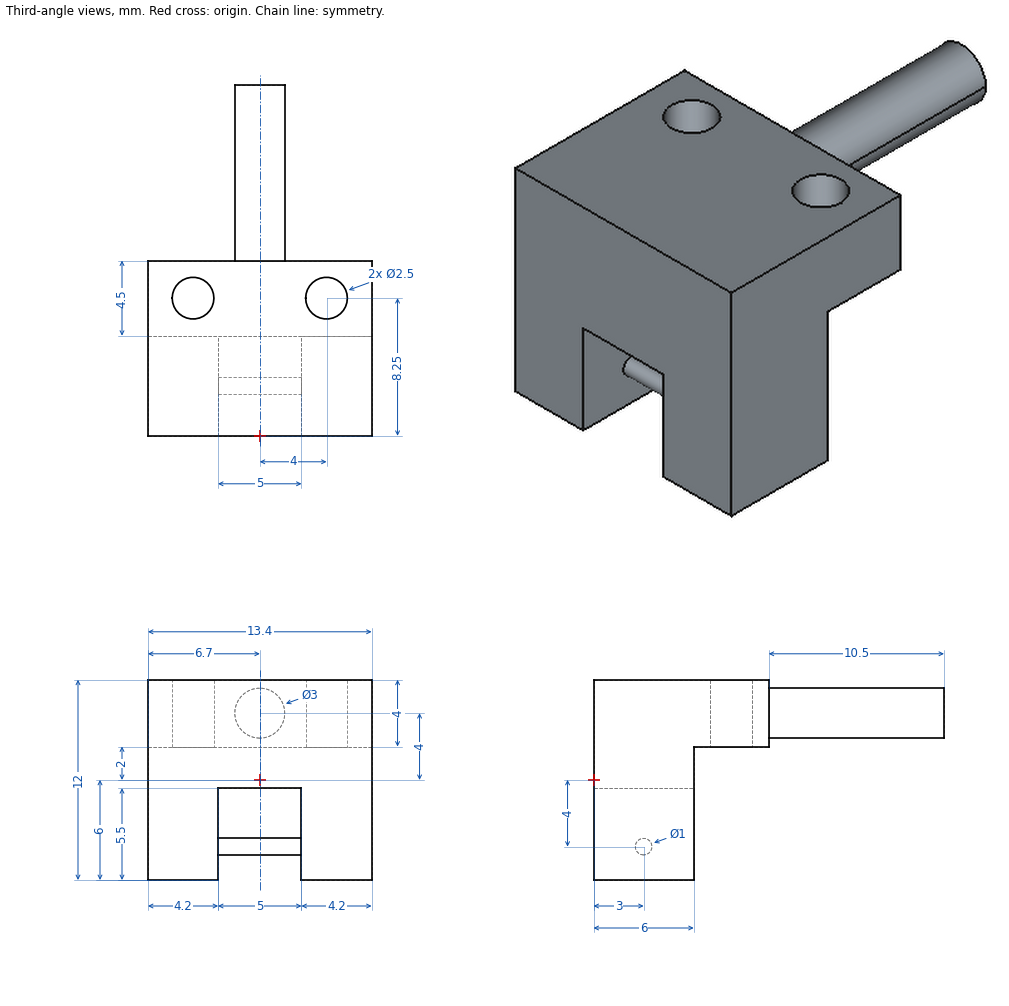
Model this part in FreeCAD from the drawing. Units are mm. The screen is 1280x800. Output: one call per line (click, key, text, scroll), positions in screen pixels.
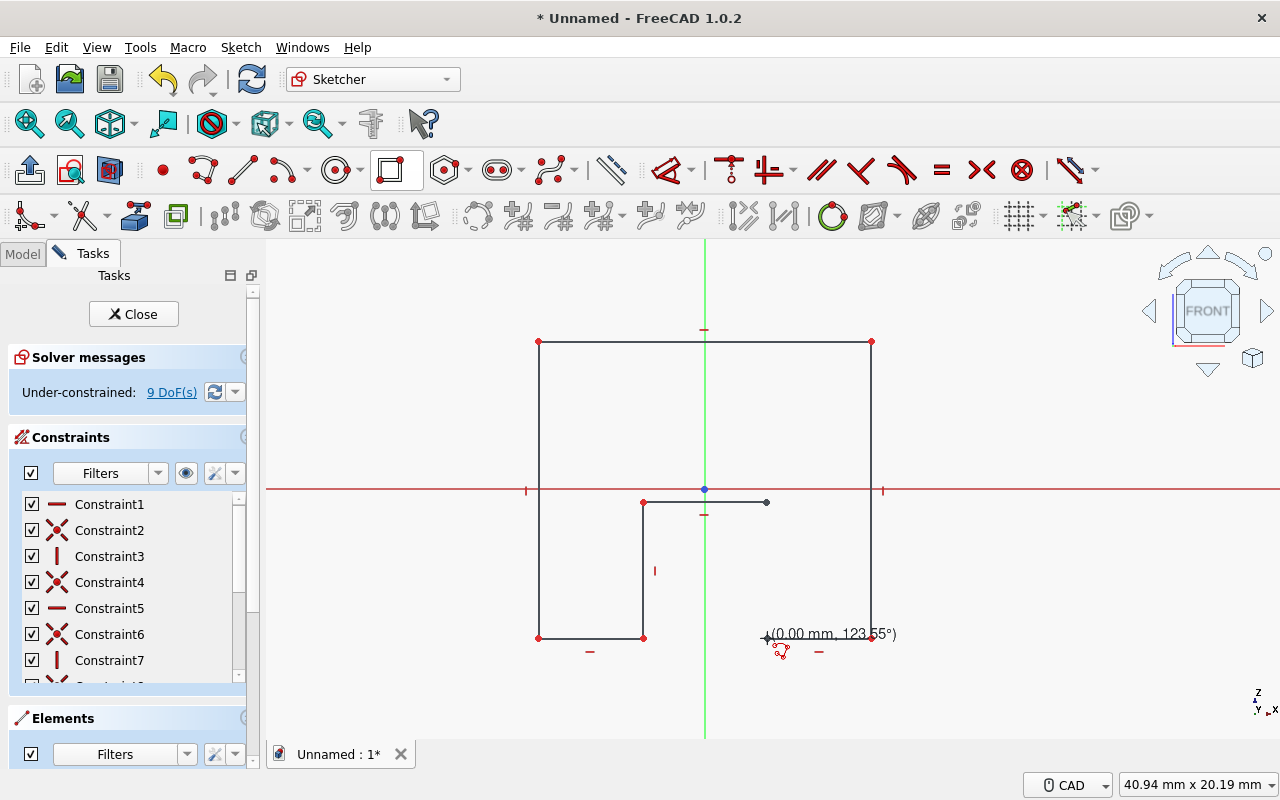
scroll(767, 502, up, 2)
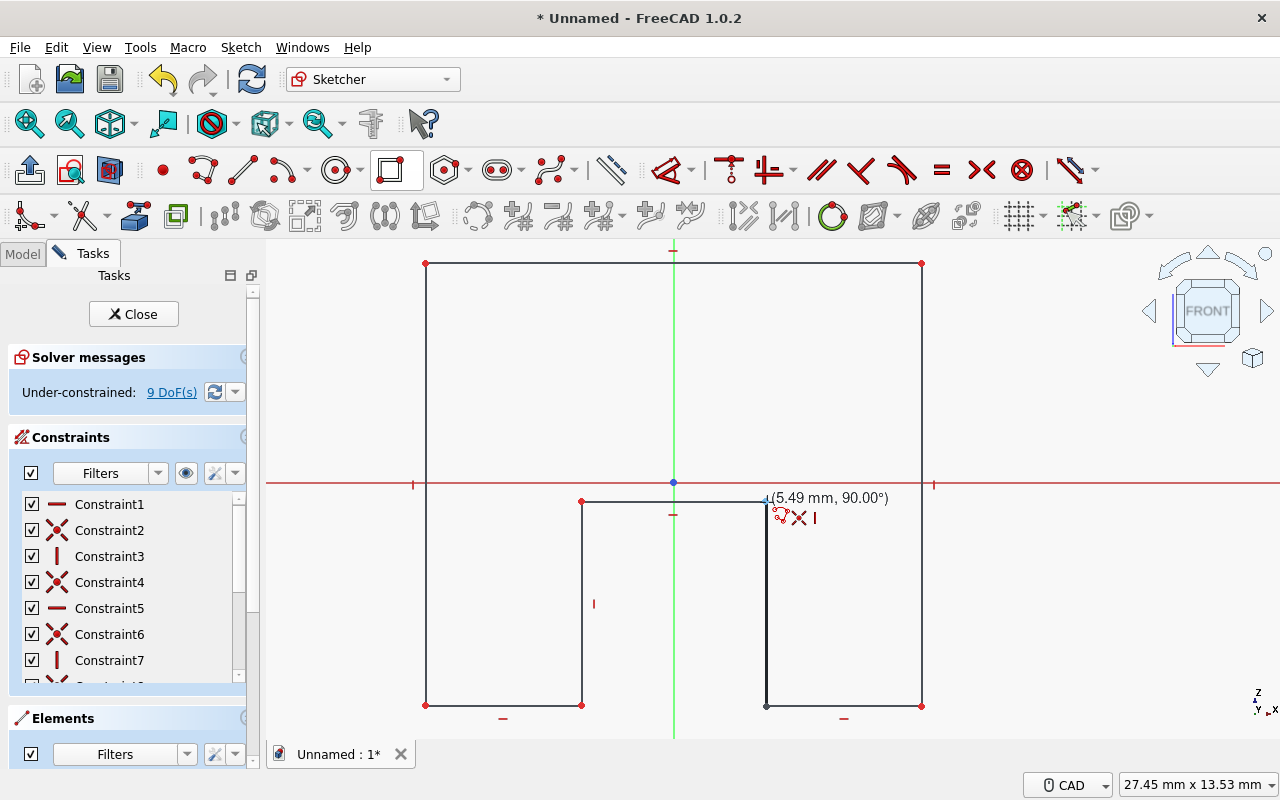
click(766, 502)
key(Escape)
key(Escape)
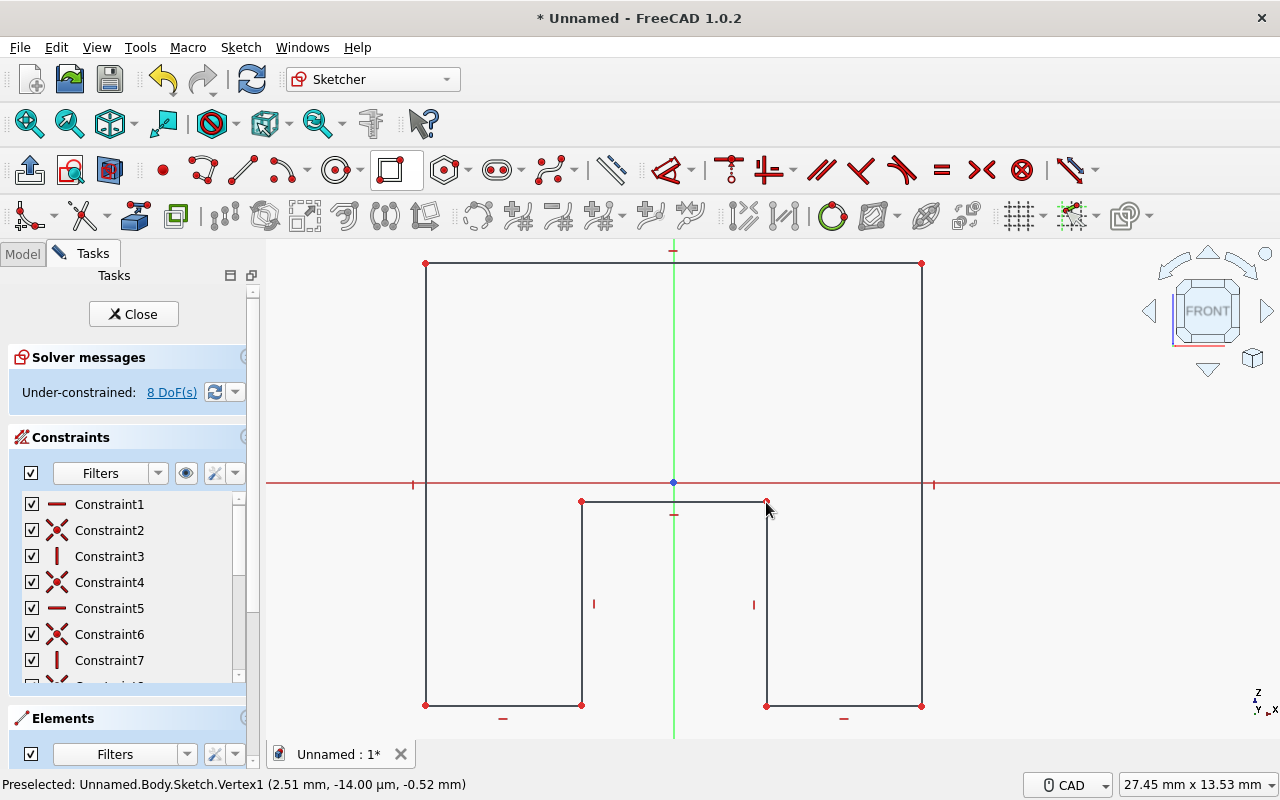
click(426, 706)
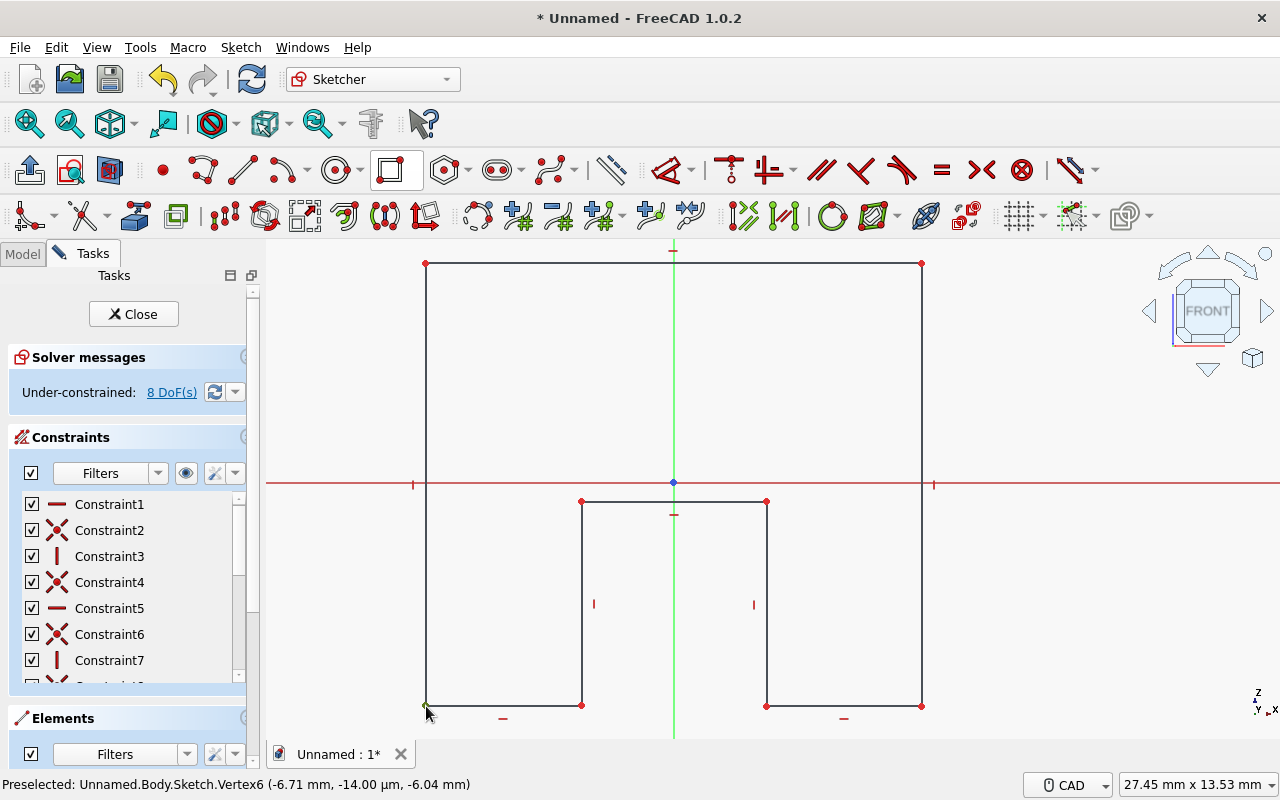
click(922, 706)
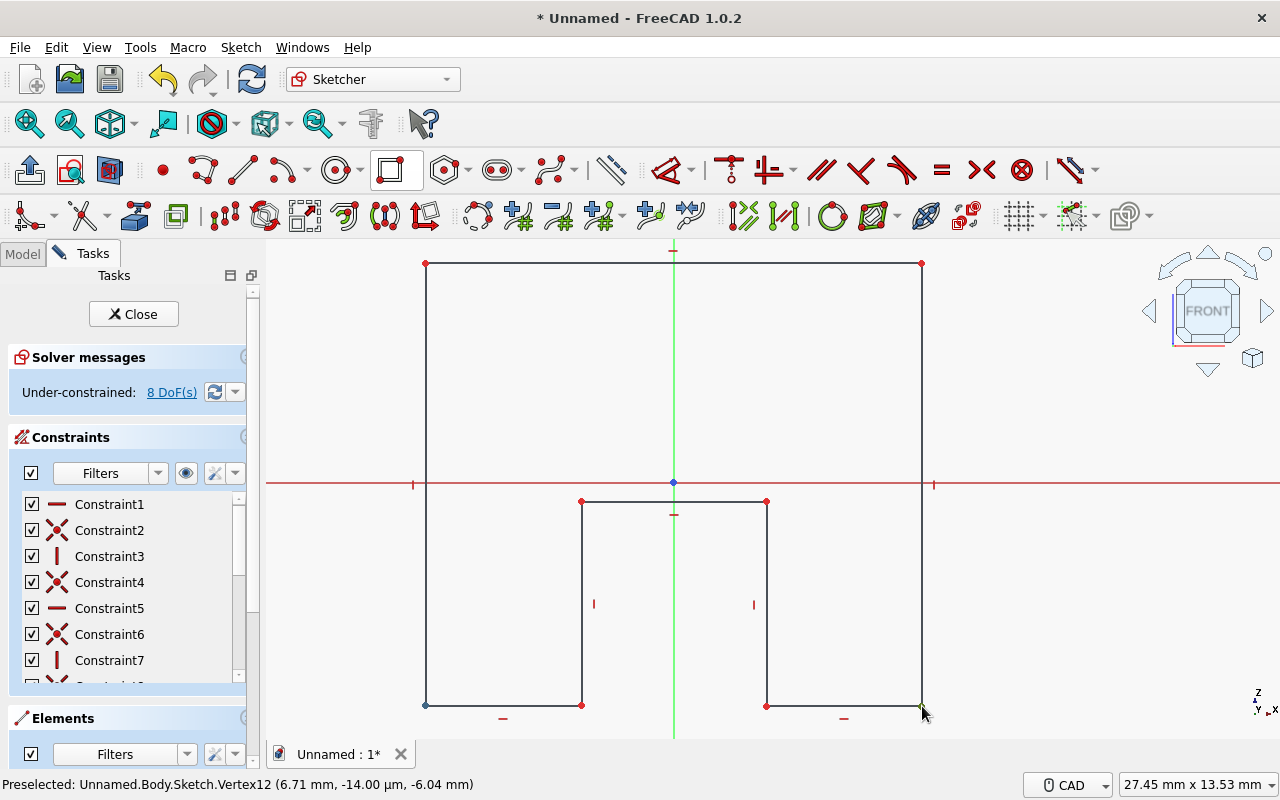
click(674, 679)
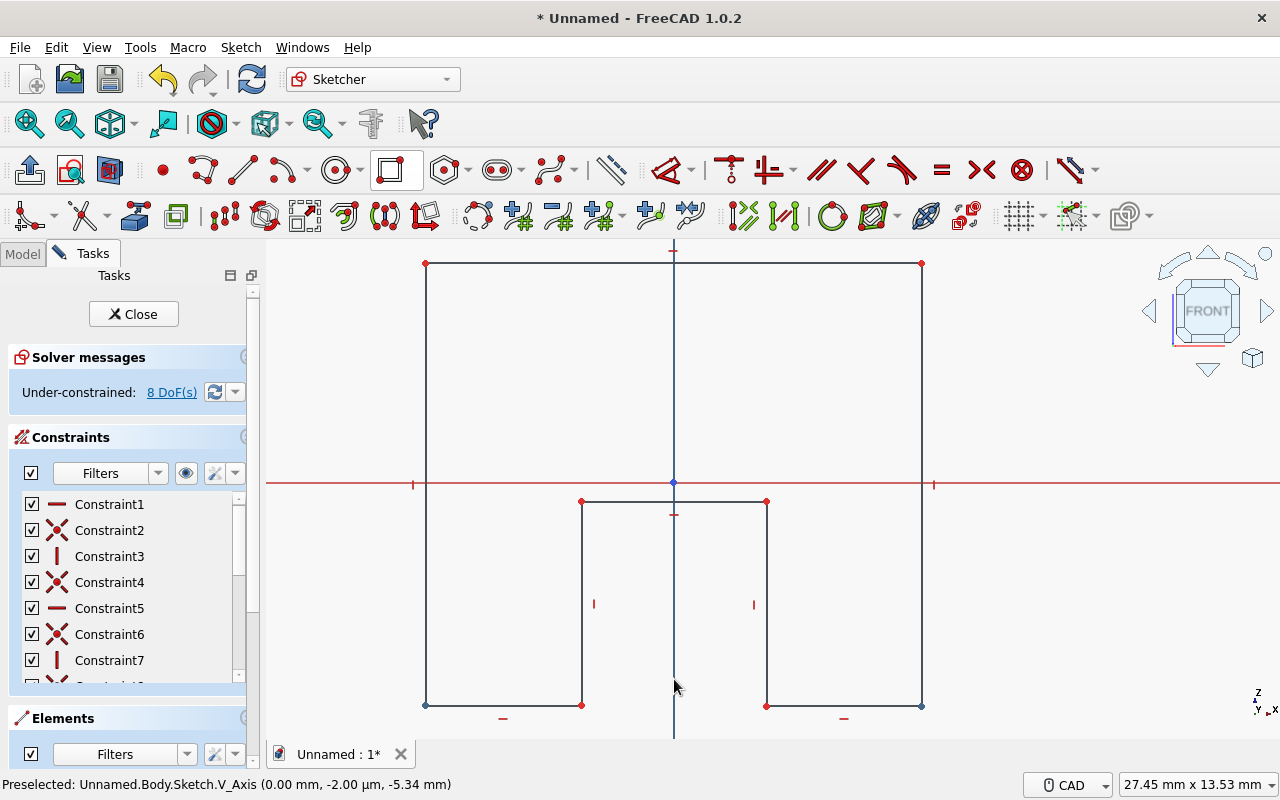
click(982, 170)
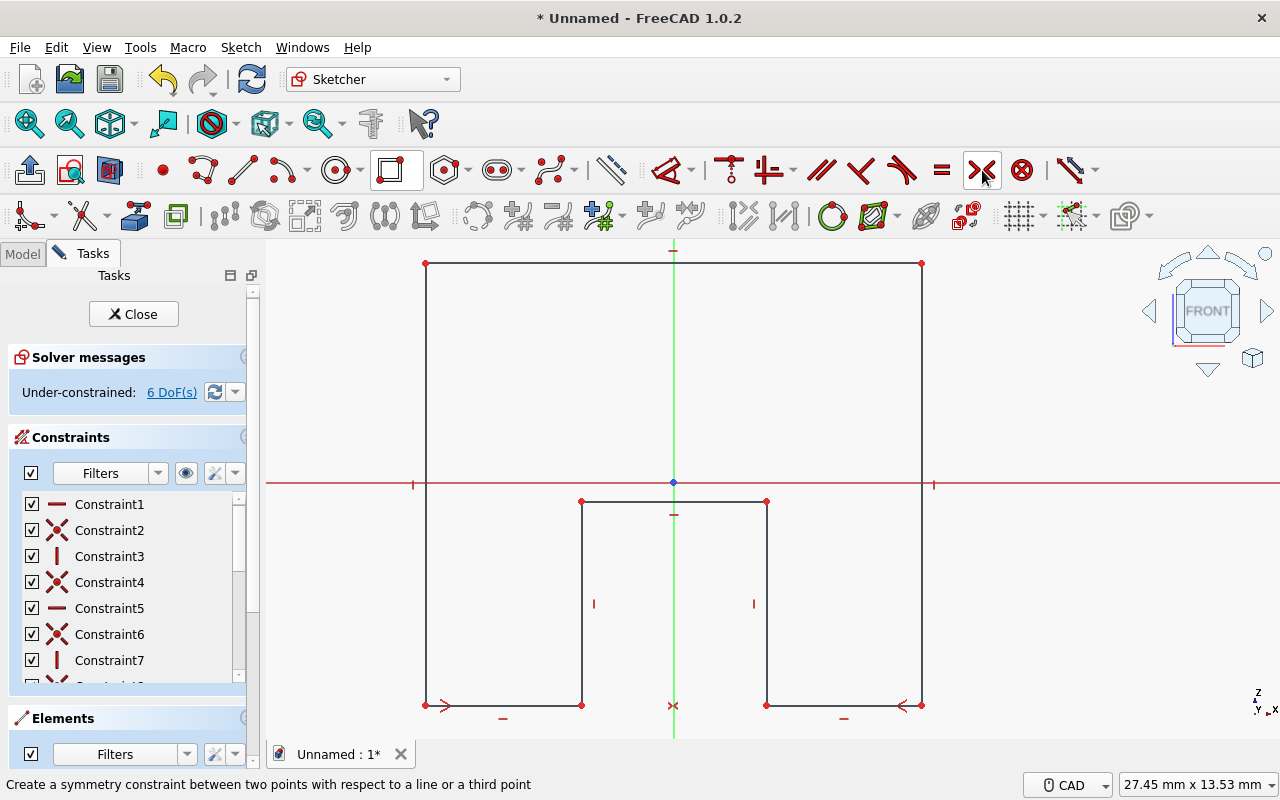
click(666, 170)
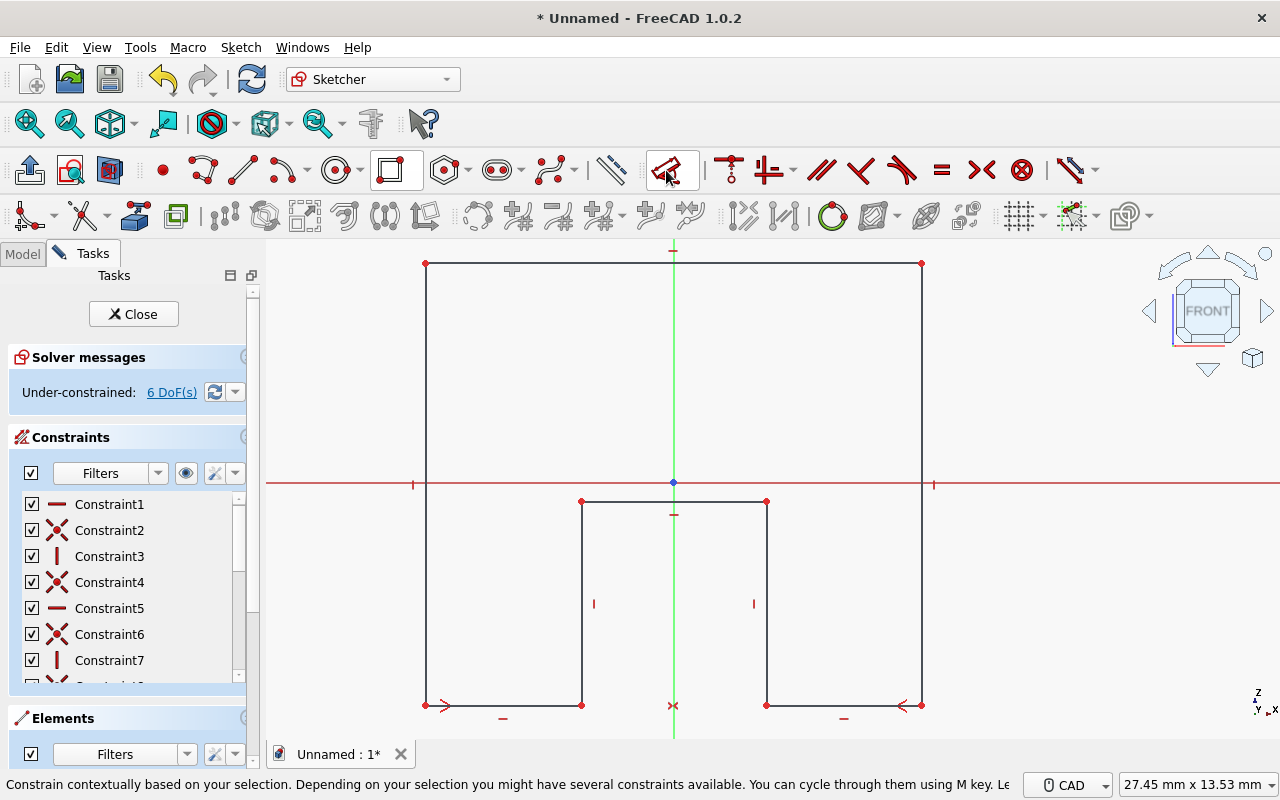
click(711, 502)
click(632, 536)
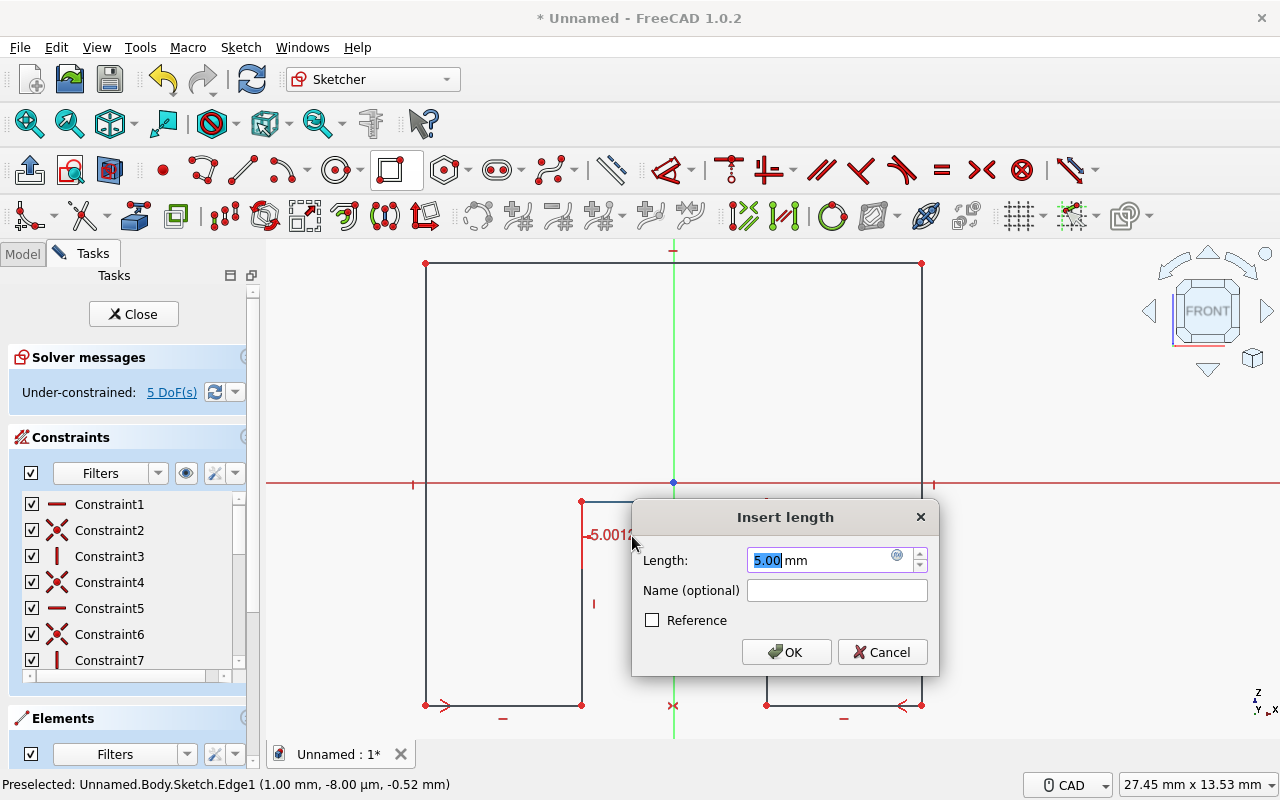
text(5)
key(Return)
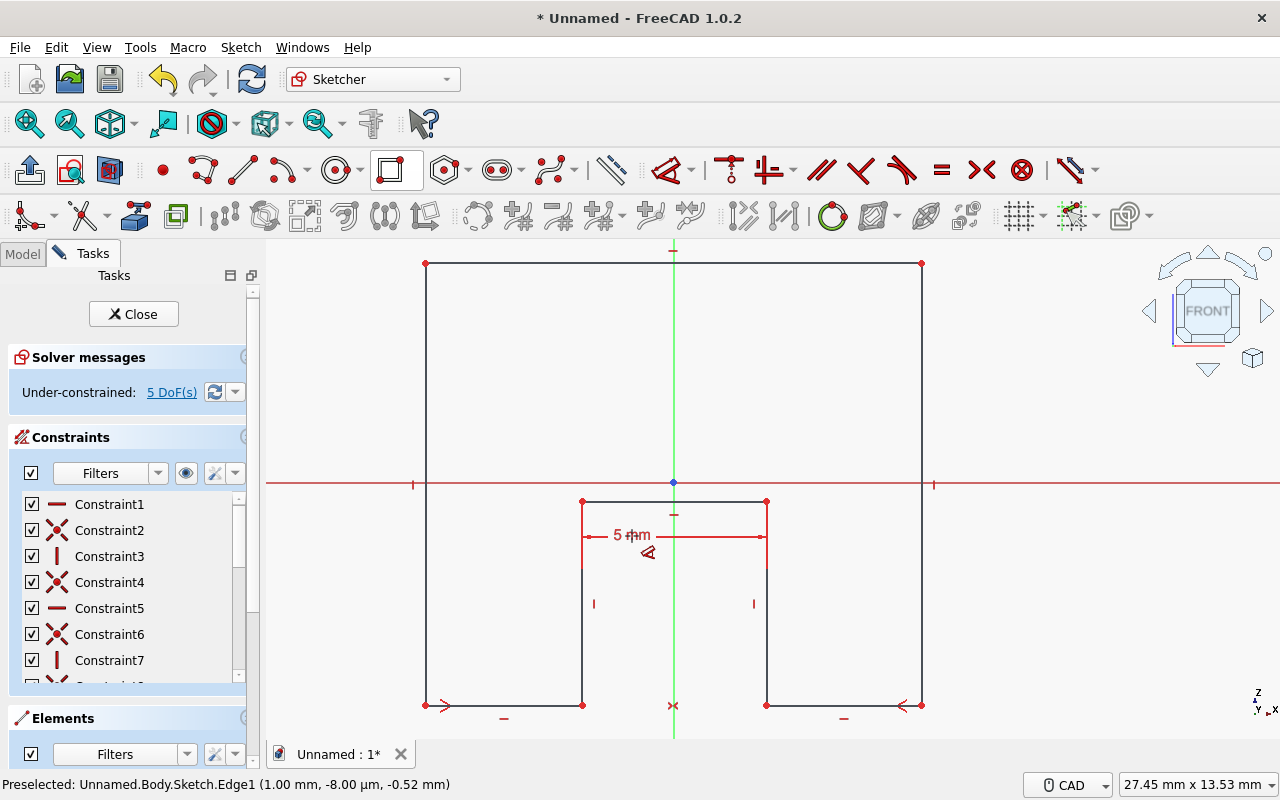
click(426, 573)
click(392, 386)